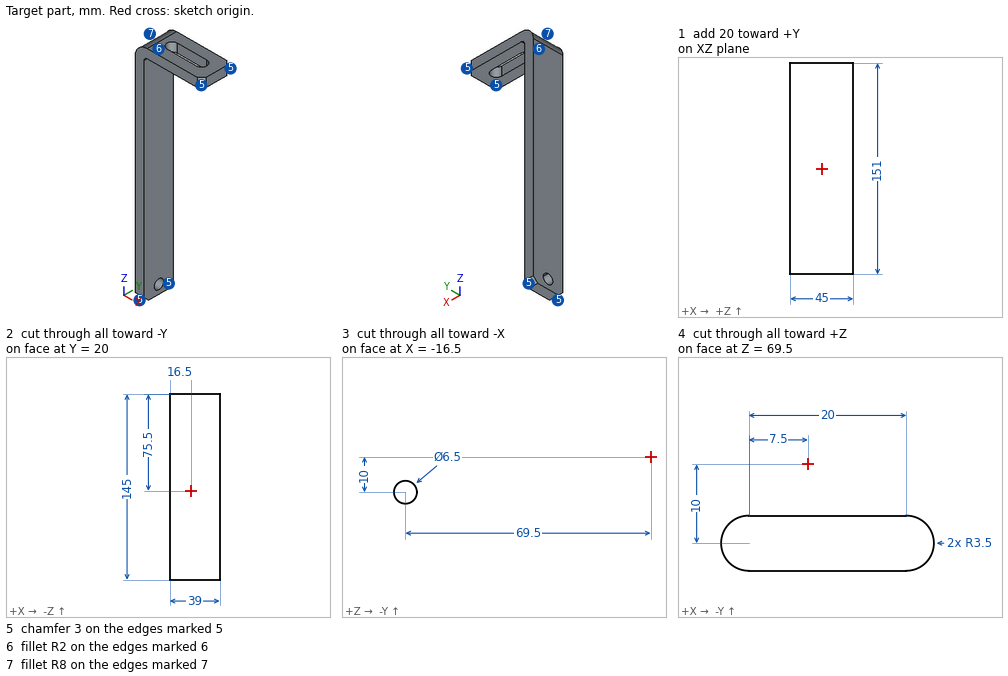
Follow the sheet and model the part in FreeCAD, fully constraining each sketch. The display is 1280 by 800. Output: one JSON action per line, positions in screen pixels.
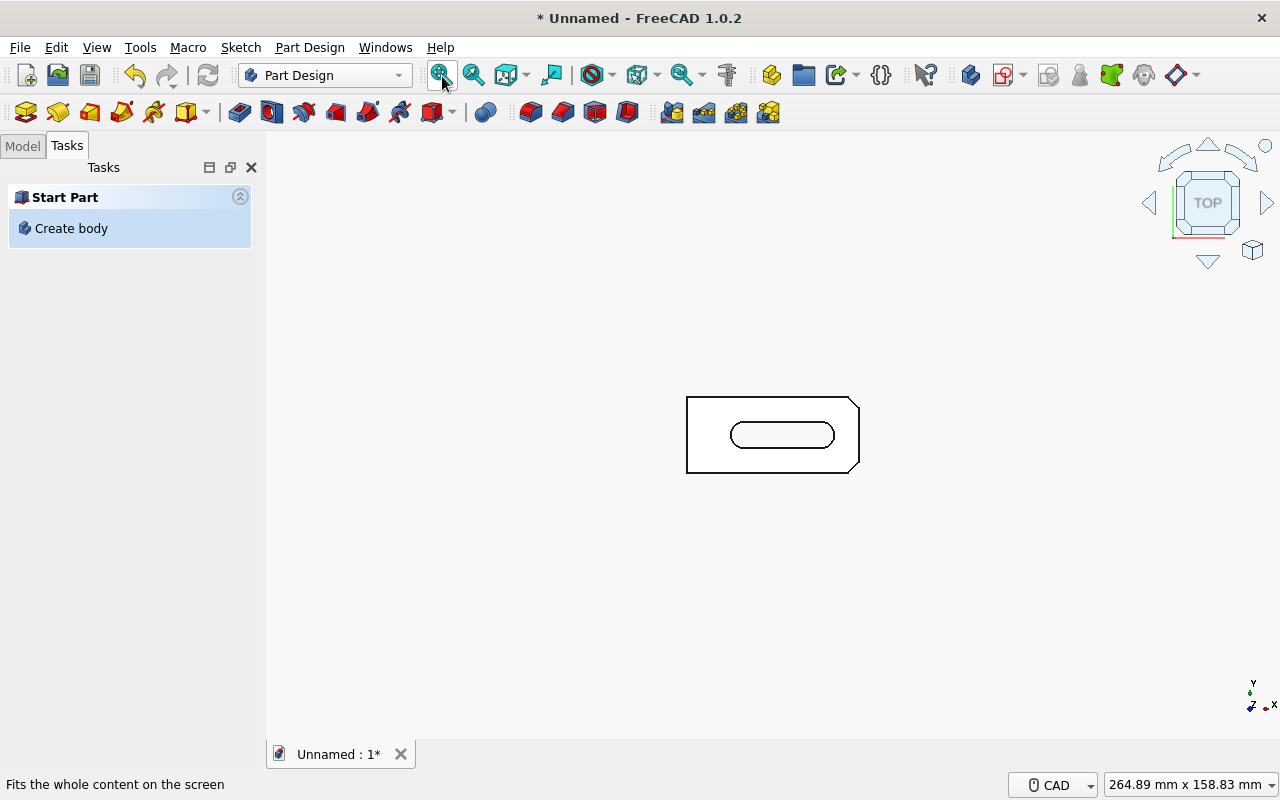
{"action": "key", "text": "0"}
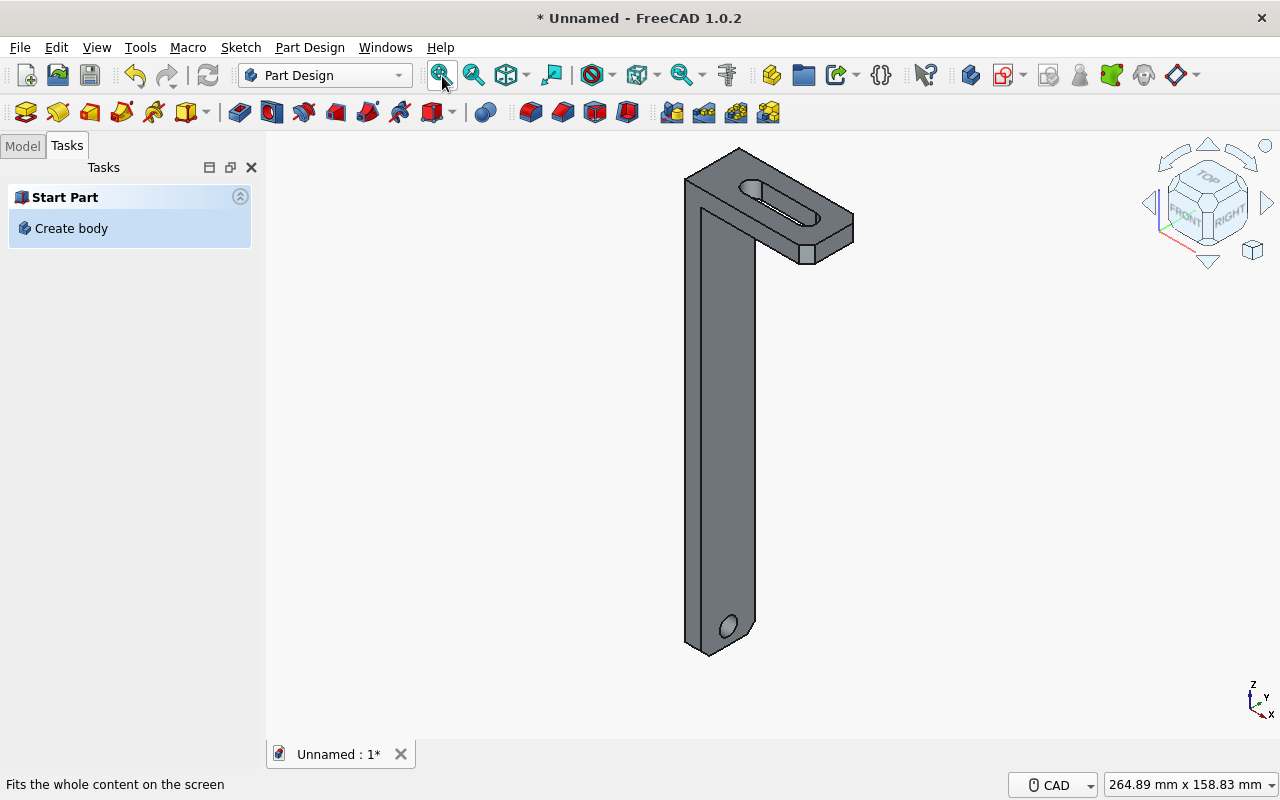
{"action": "key", "text": "1"}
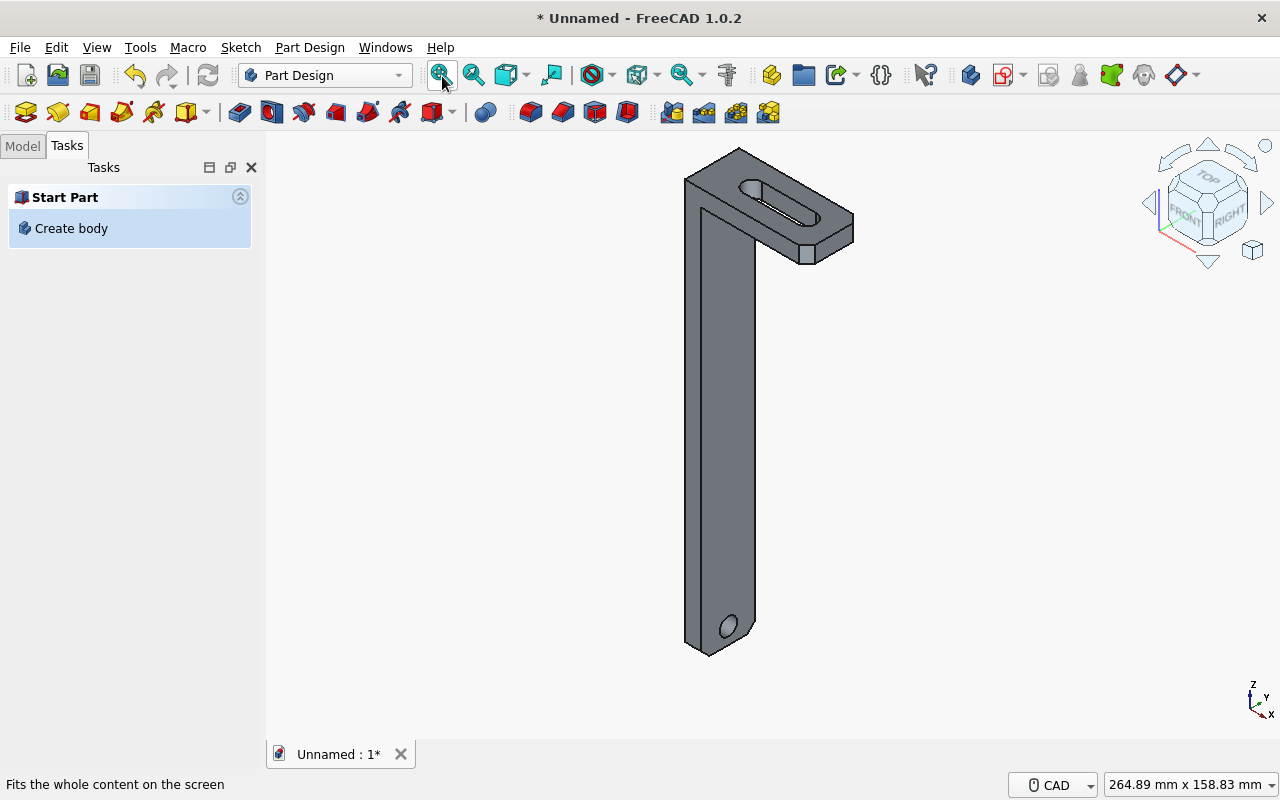
{"action": "key", "text": "3"}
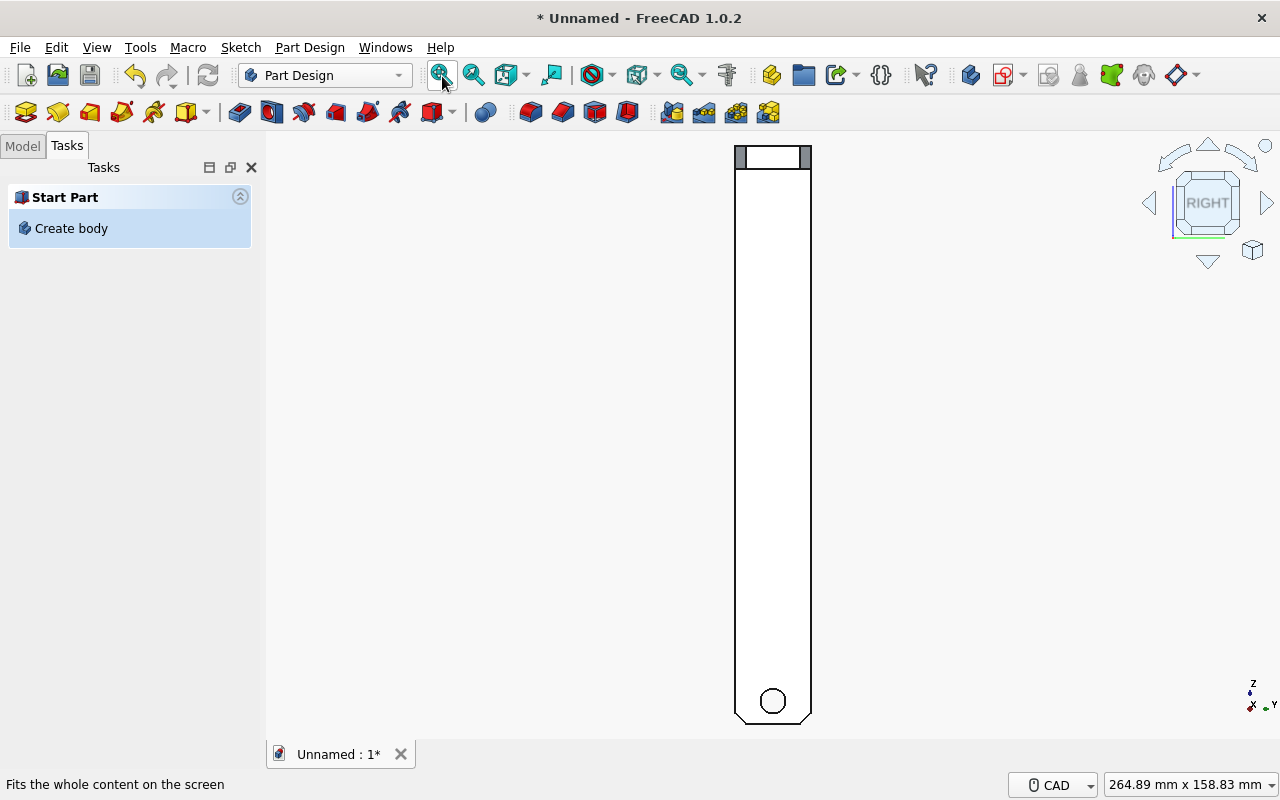
{"action": "key", "text": "5"}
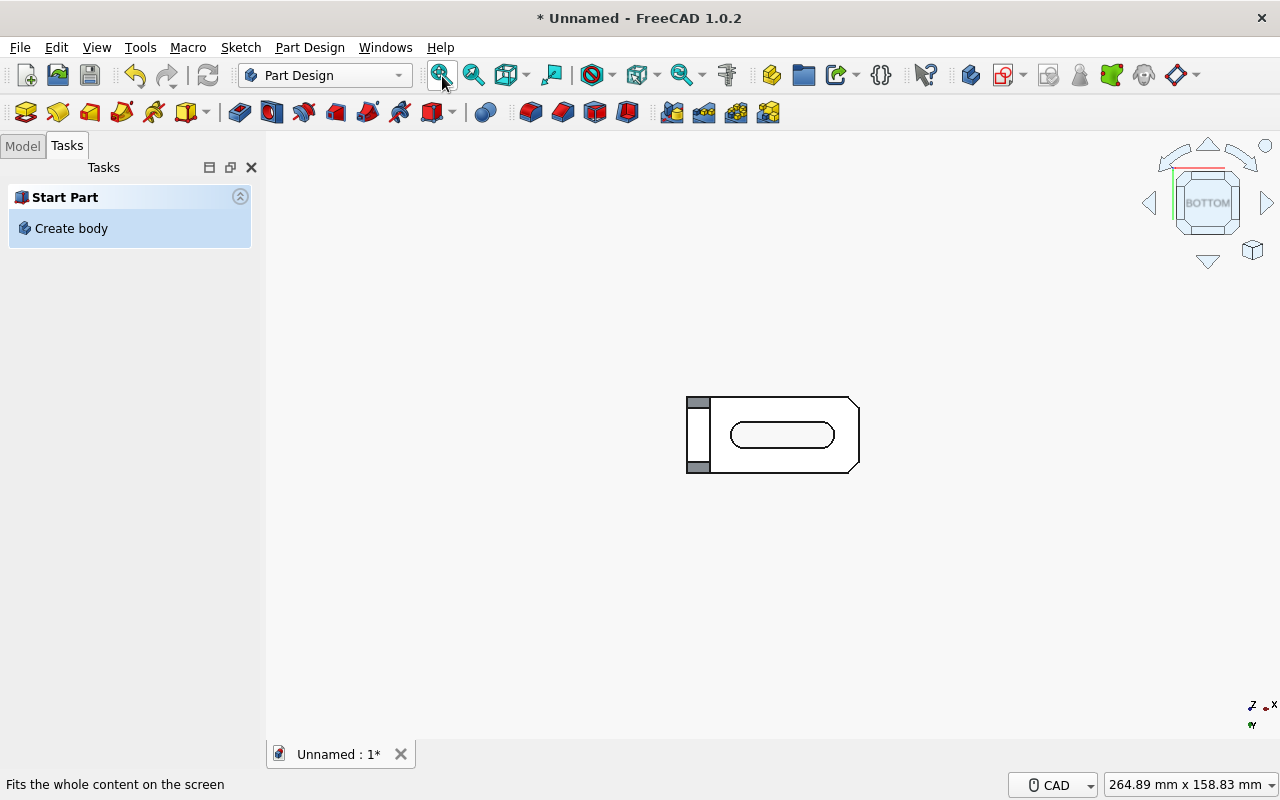
{"action": "left_click", "coordinate": [442, 76]}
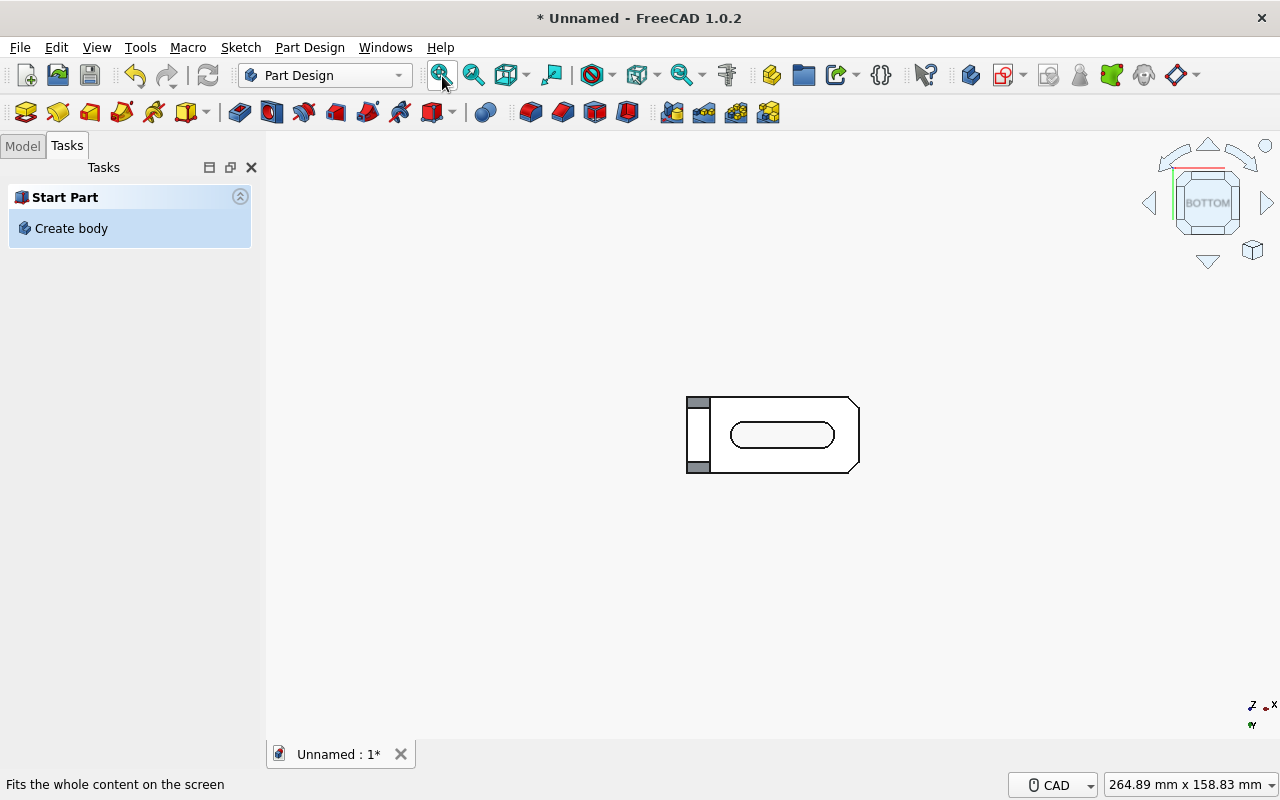
{"action": "key", "text": "4"}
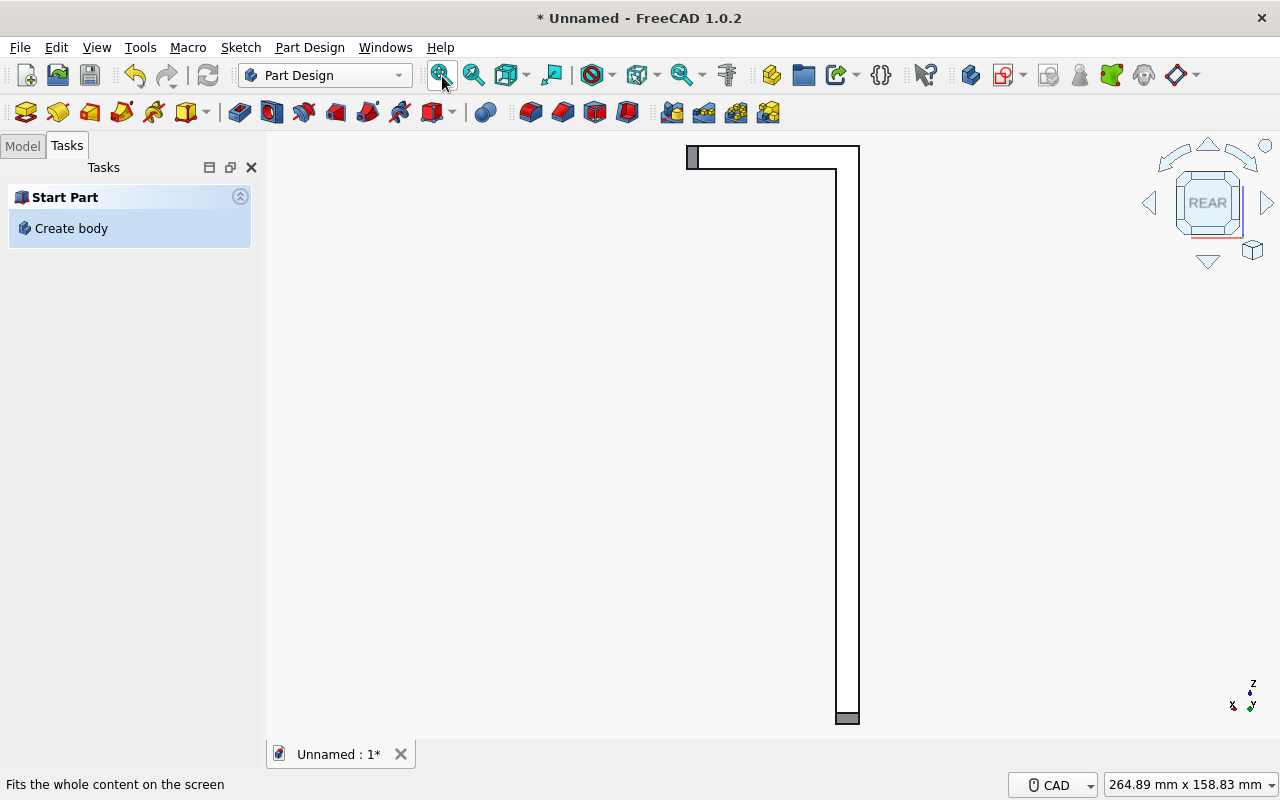
{"action": "key", "text": "6"}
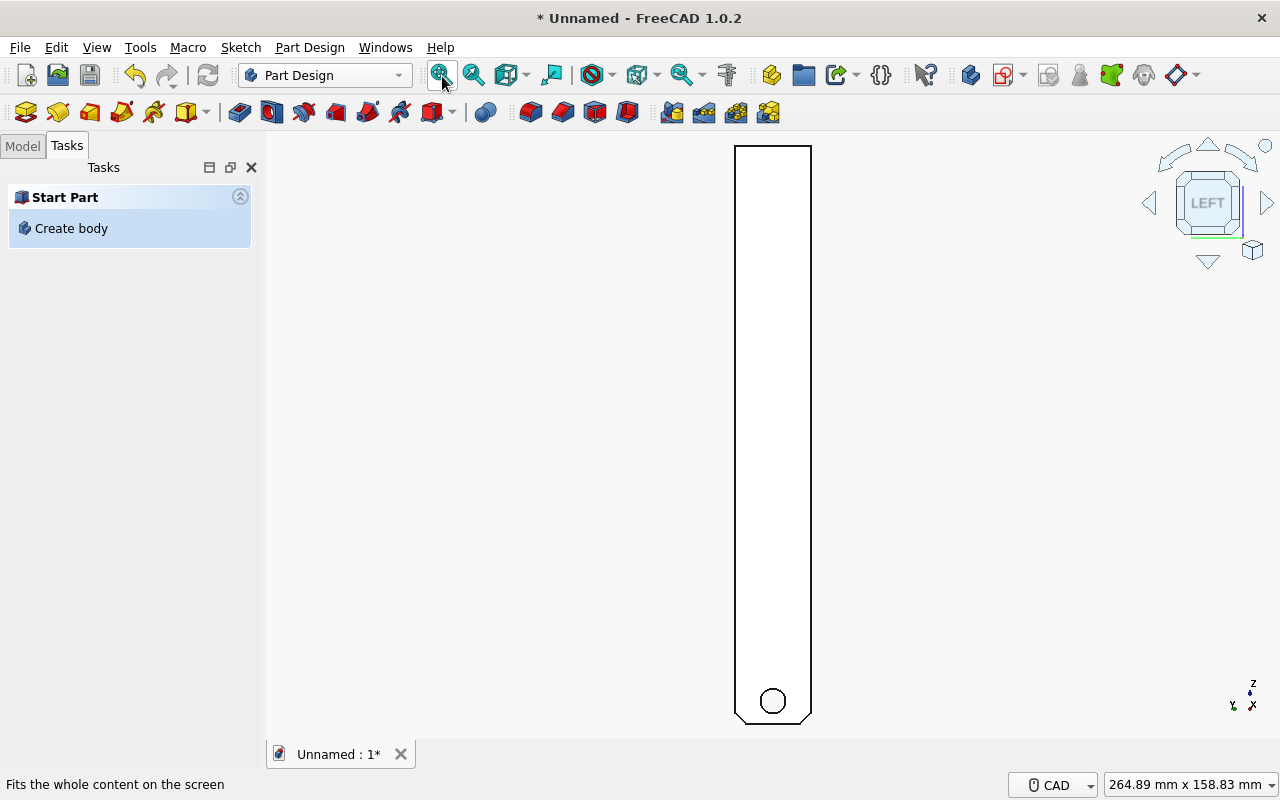
{"action": "key", "text": "v 3"}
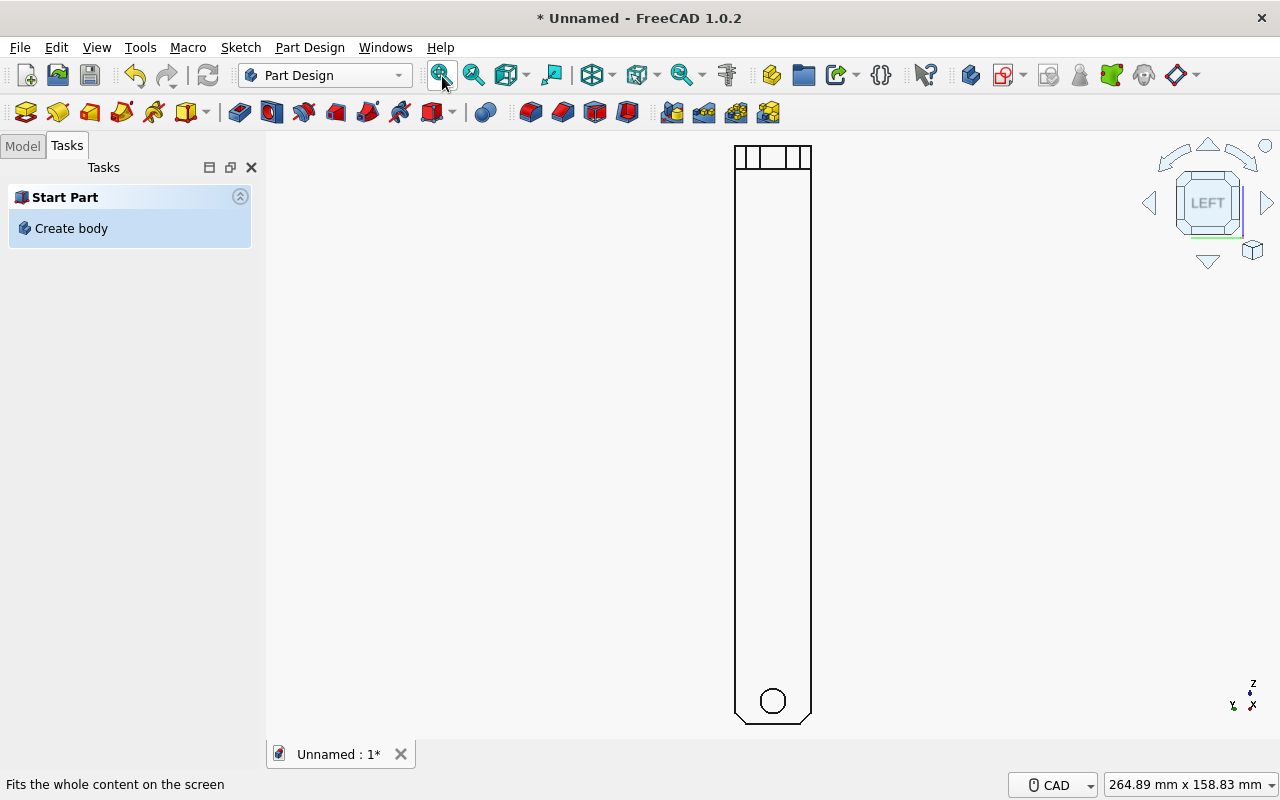
{"action": "key", "text": "0"}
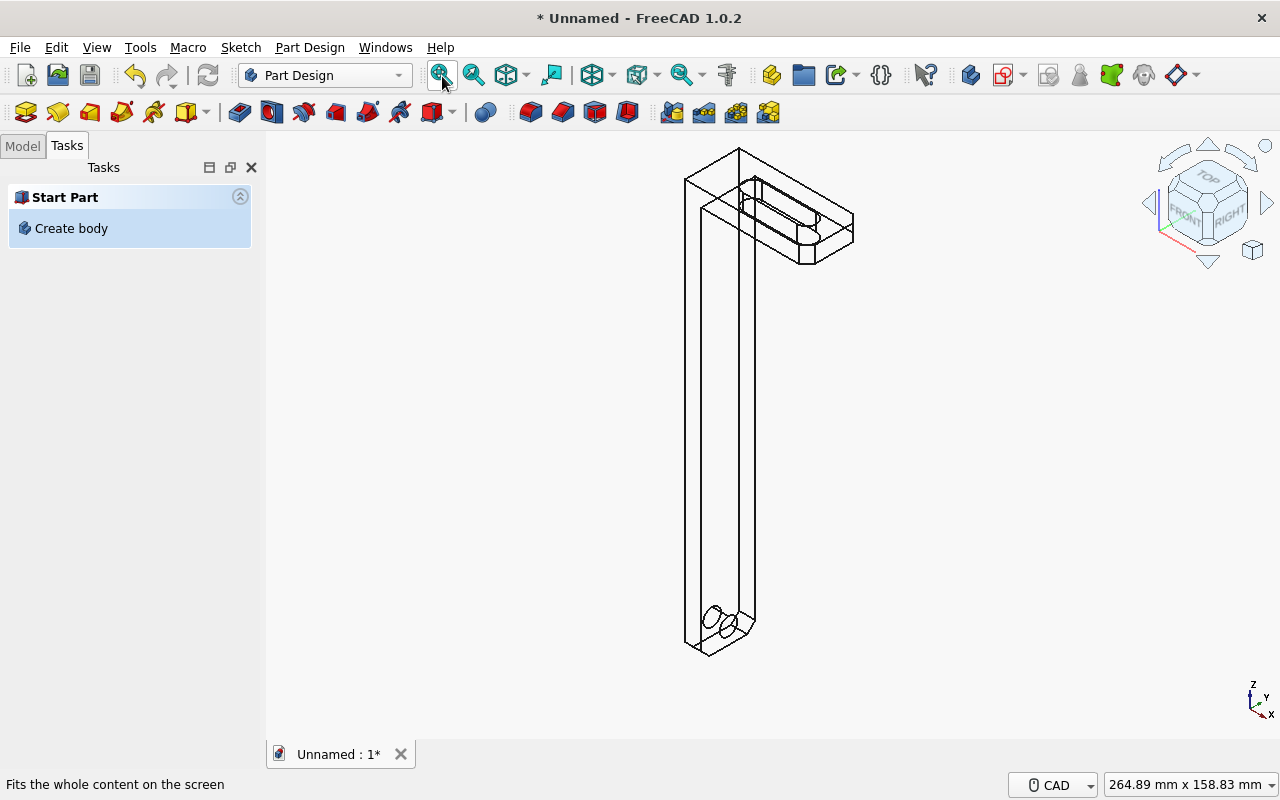
{"action": "left_click", "coordinate": [728, 191]}